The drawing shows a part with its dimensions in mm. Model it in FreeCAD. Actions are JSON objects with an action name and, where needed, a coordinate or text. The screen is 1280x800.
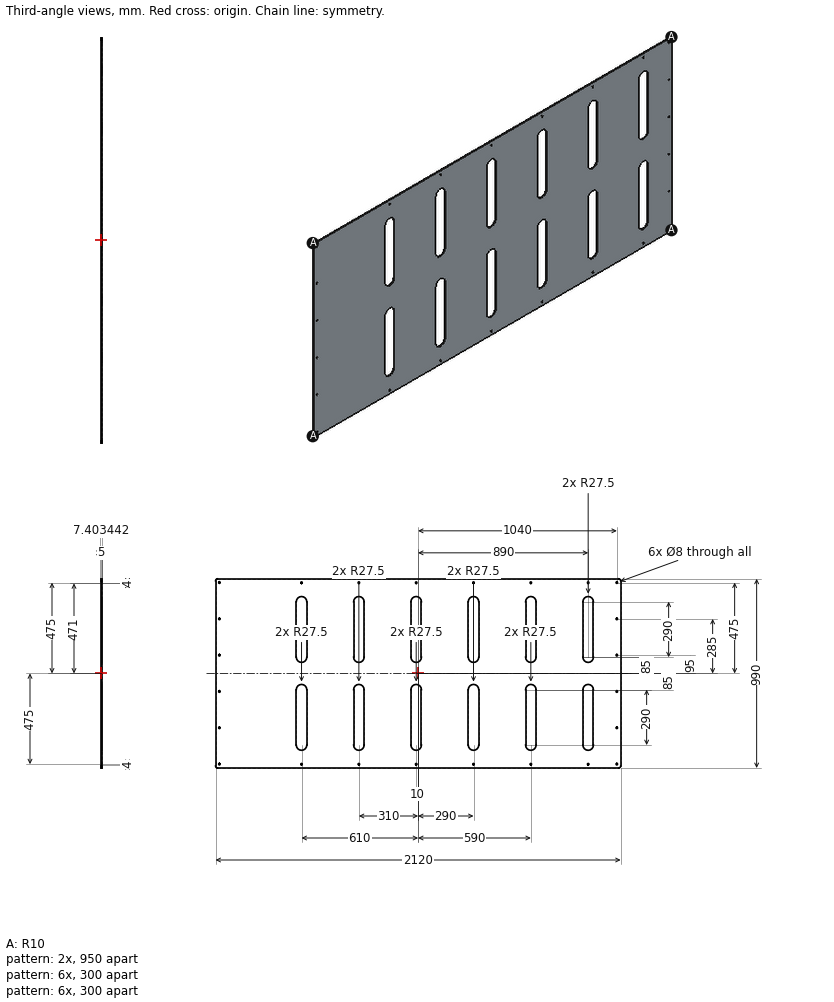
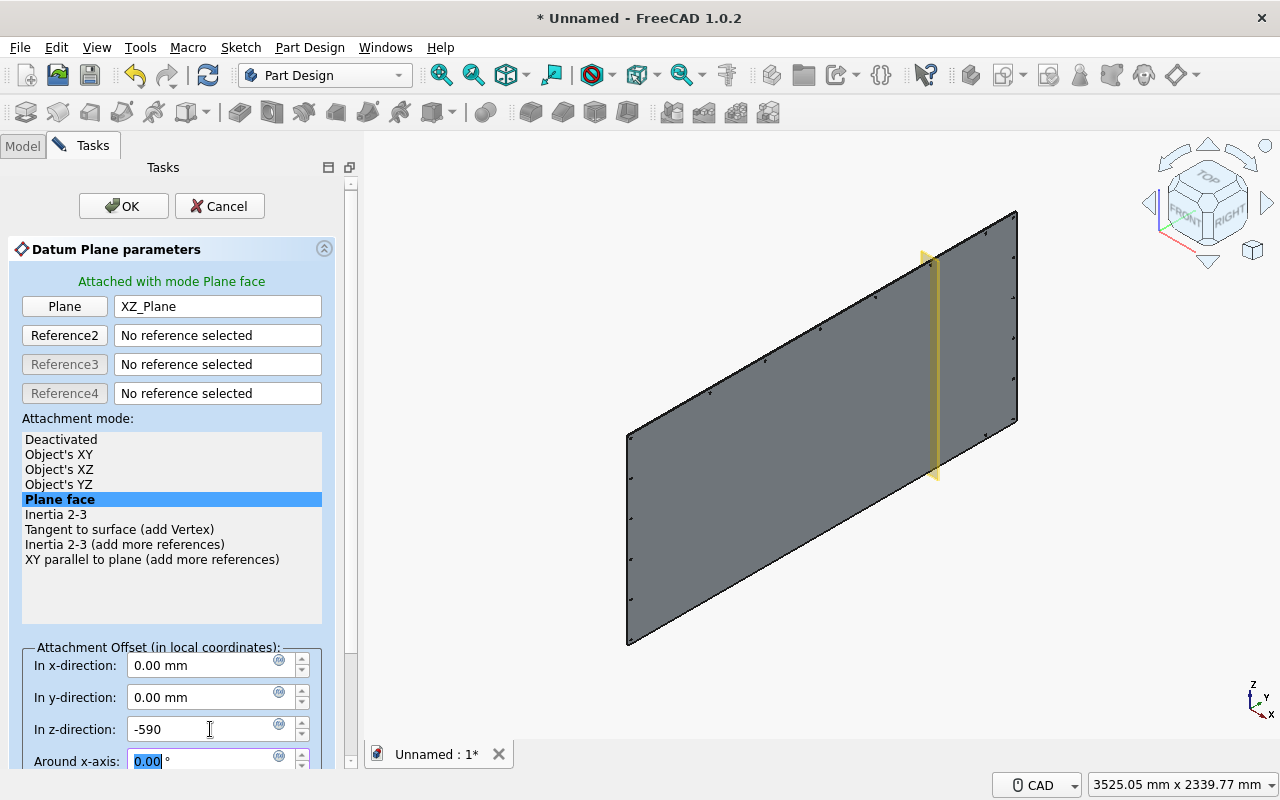
{"action": "left_click", "coordinate": [124, 206]}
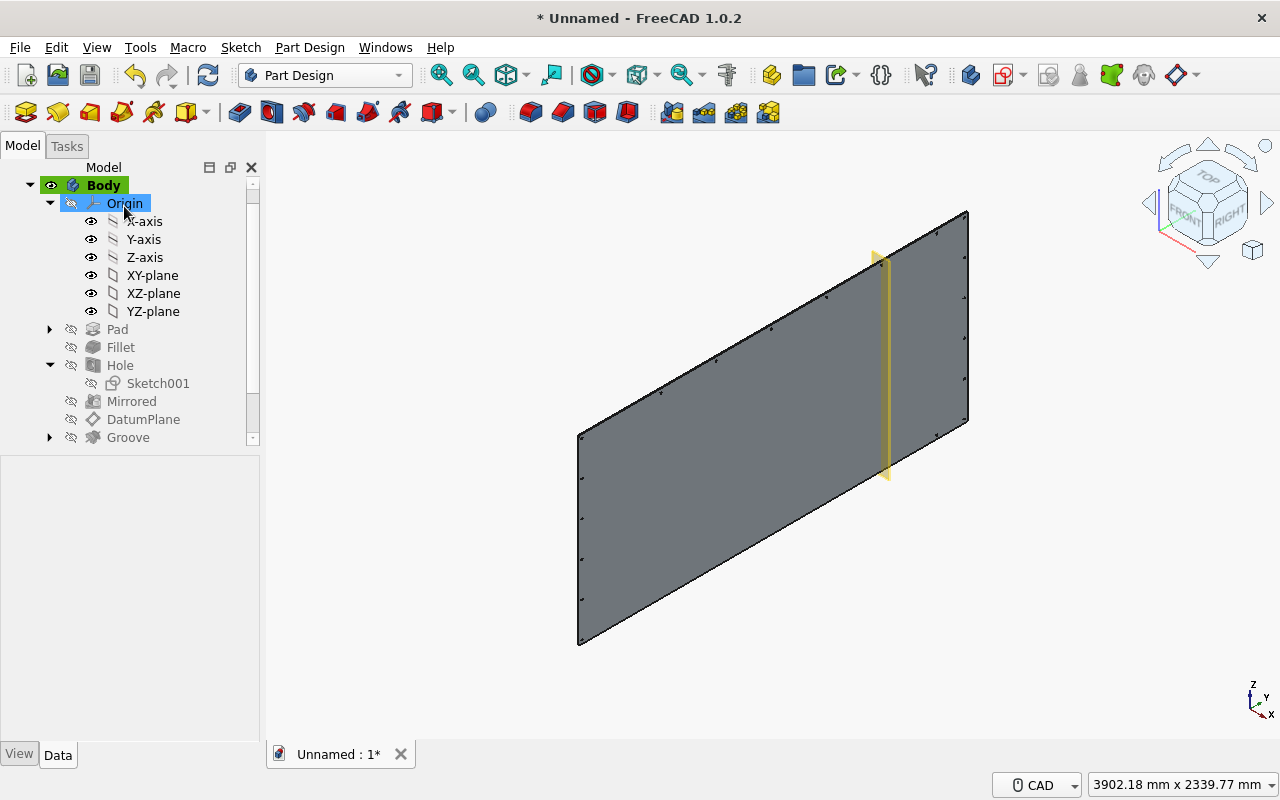
{"action": "scroll", "coordinate": [120, 307], "scroll_direction": "down", "scroll_amount": 3}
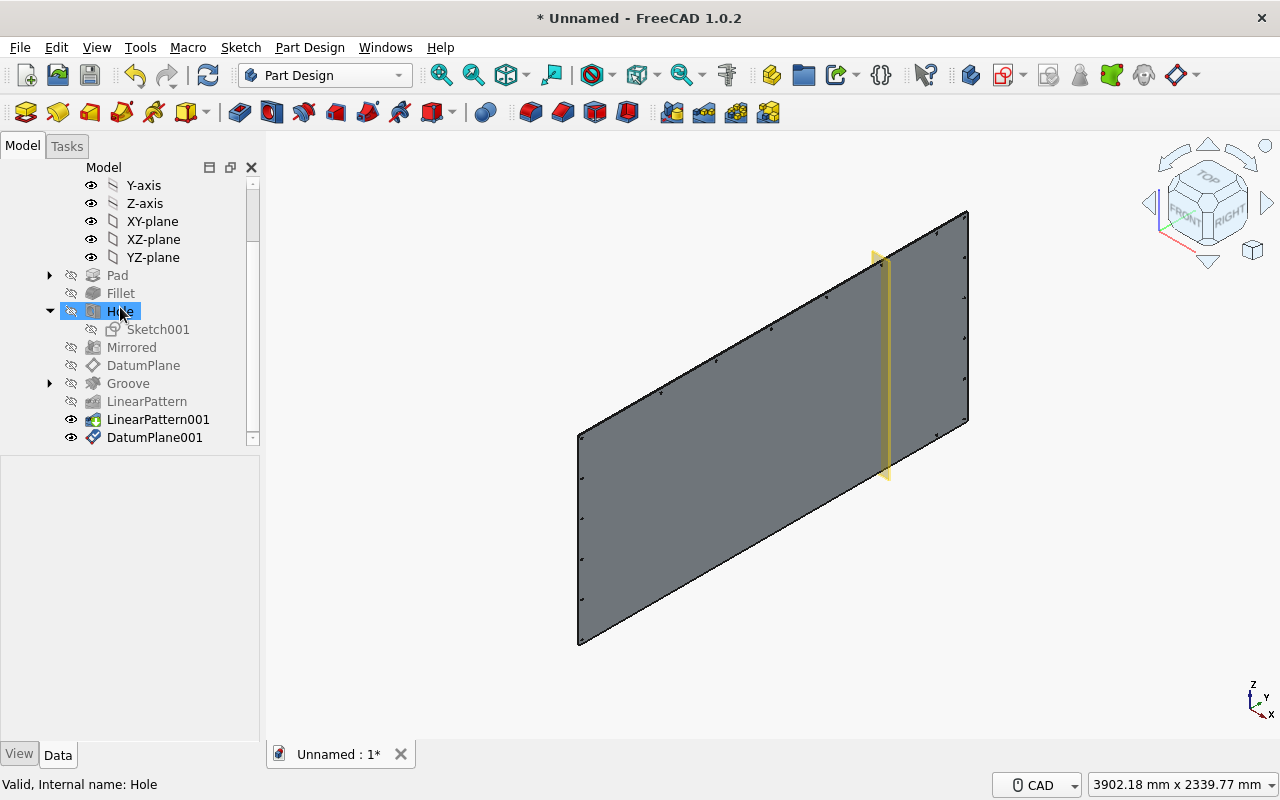
{"action": "left_click", "coordinate": [116, 437]}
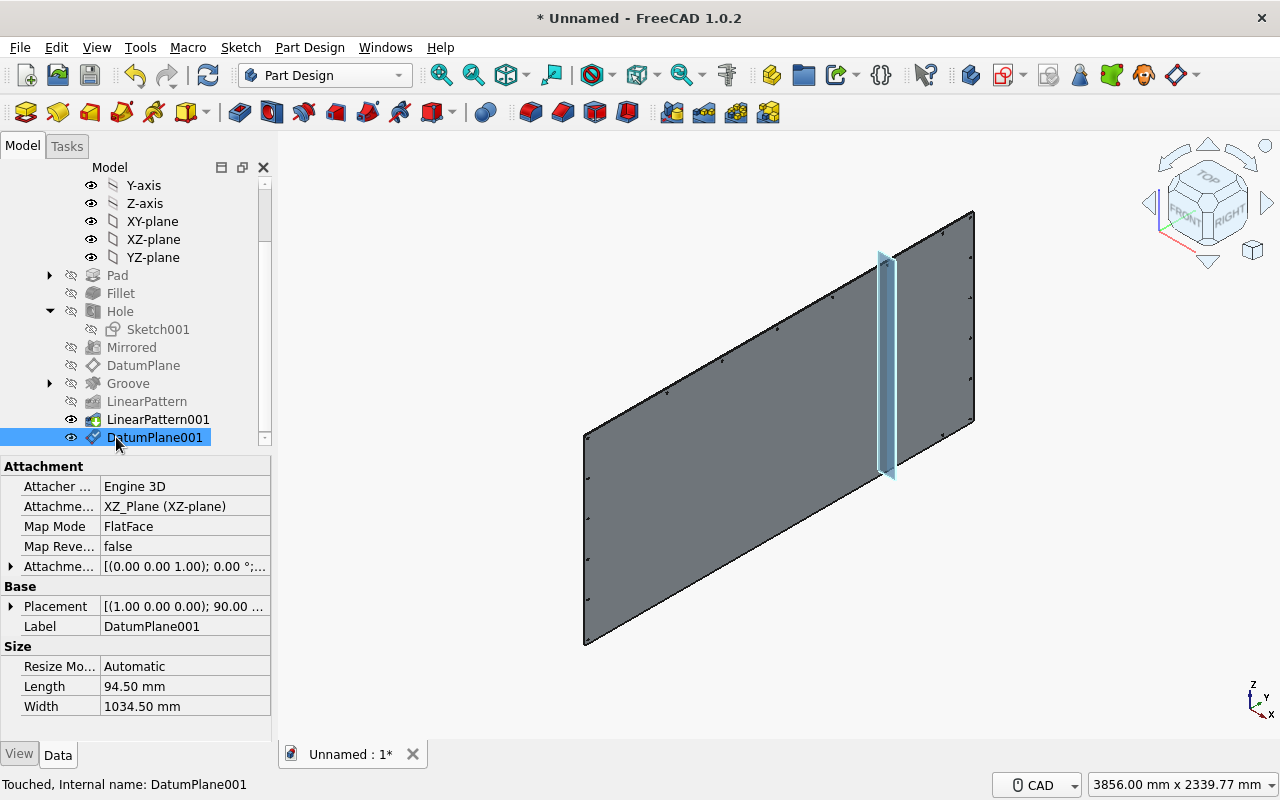
{"action": "left_click", "coordinate": [1004, 76]}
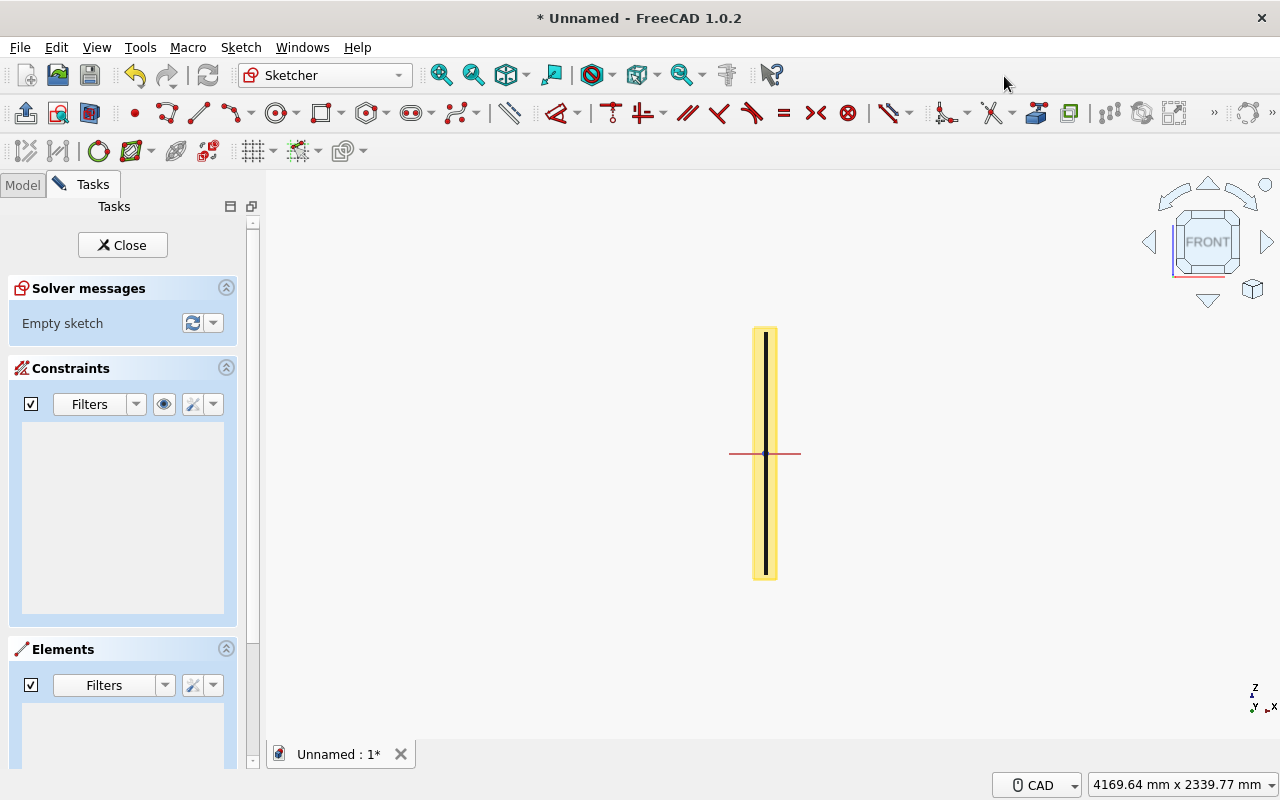
{"action": "left_click", "coordinate": [90, 114]}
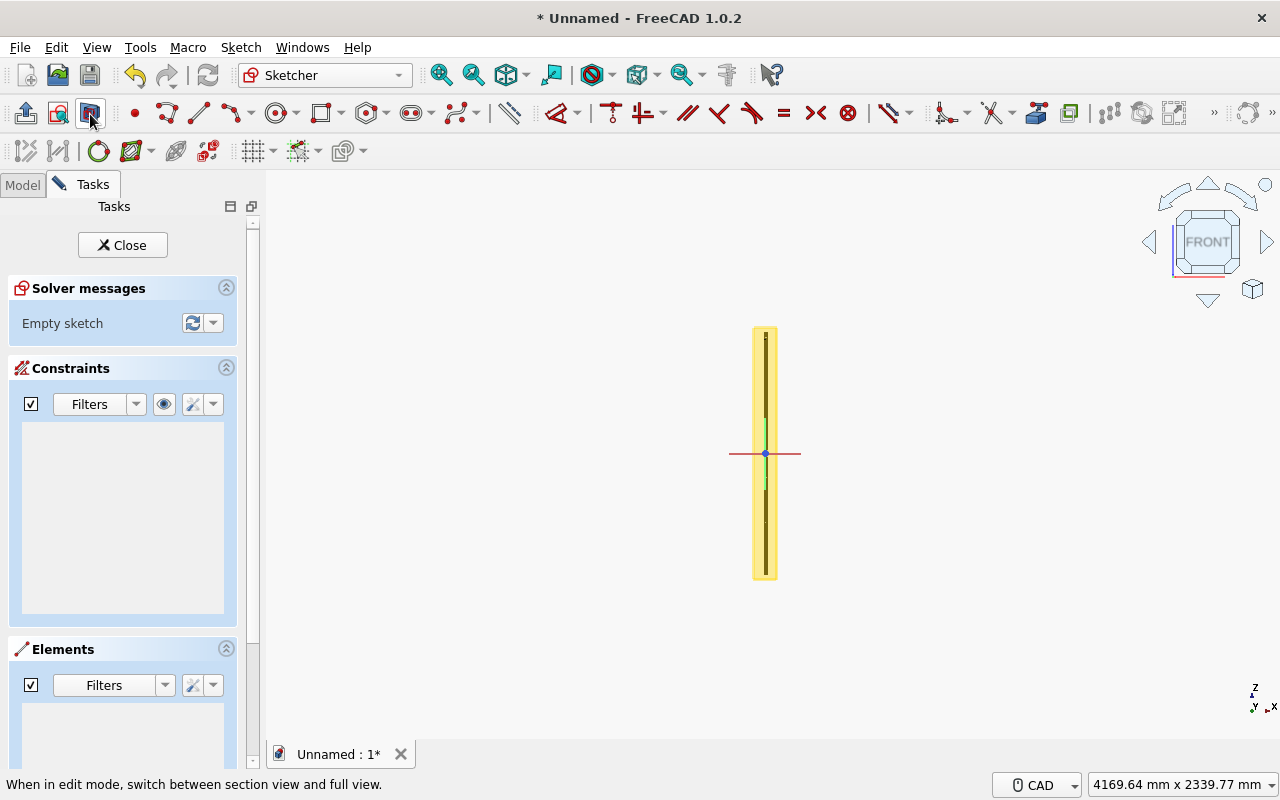
{"action": "scroll", "coordinate": [769, 576], "scroll_direction": "up", "scroll_amount": 15}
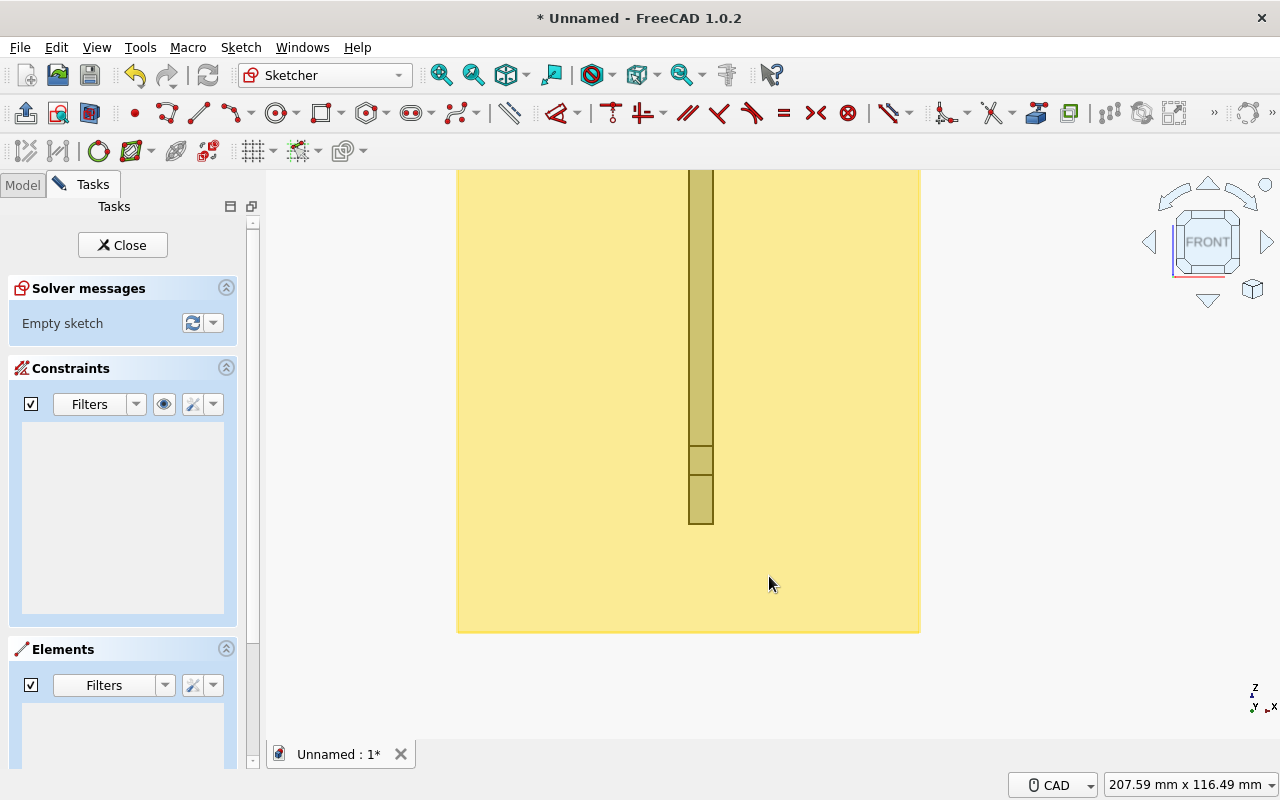
{"action": "scroll", "coordinate": [686, 434], "scroll_direction": "up", "scroll_amount": 12}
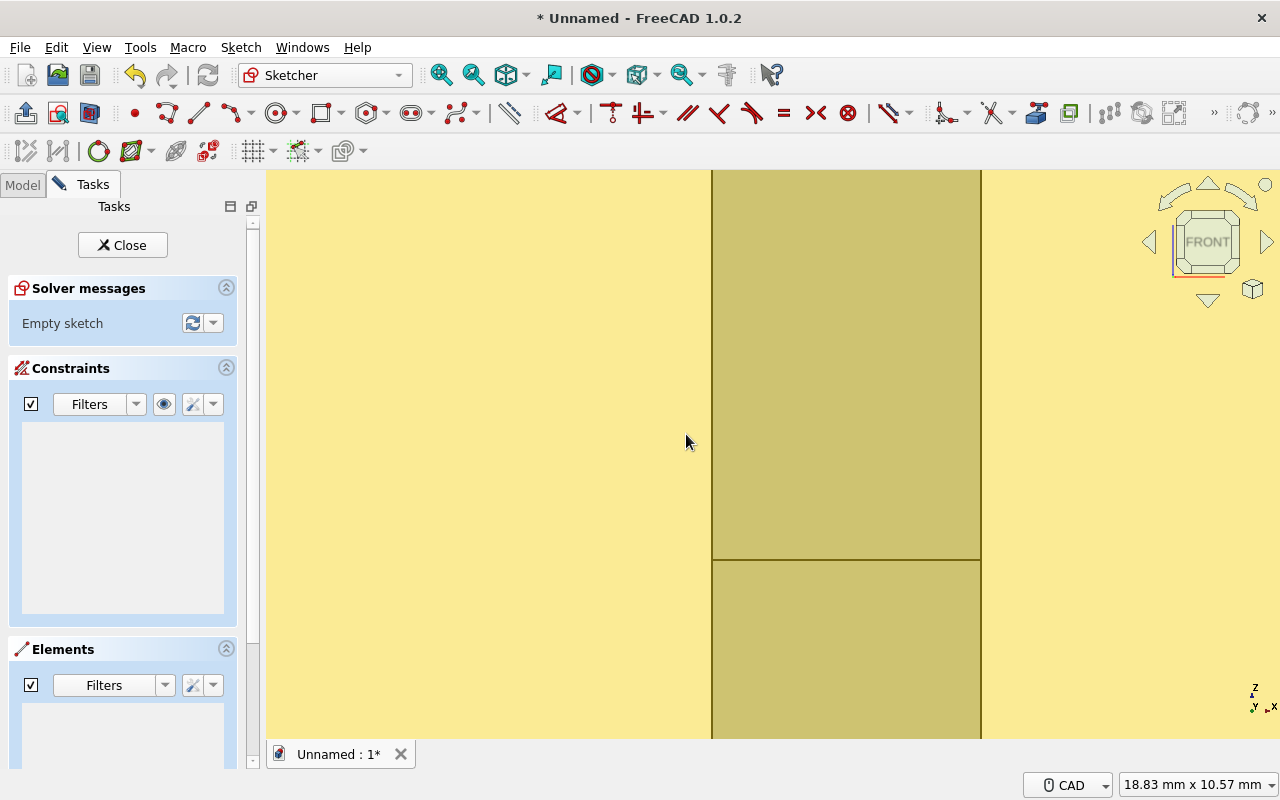
{"action": "left_click", "coordinate": [168, 114]}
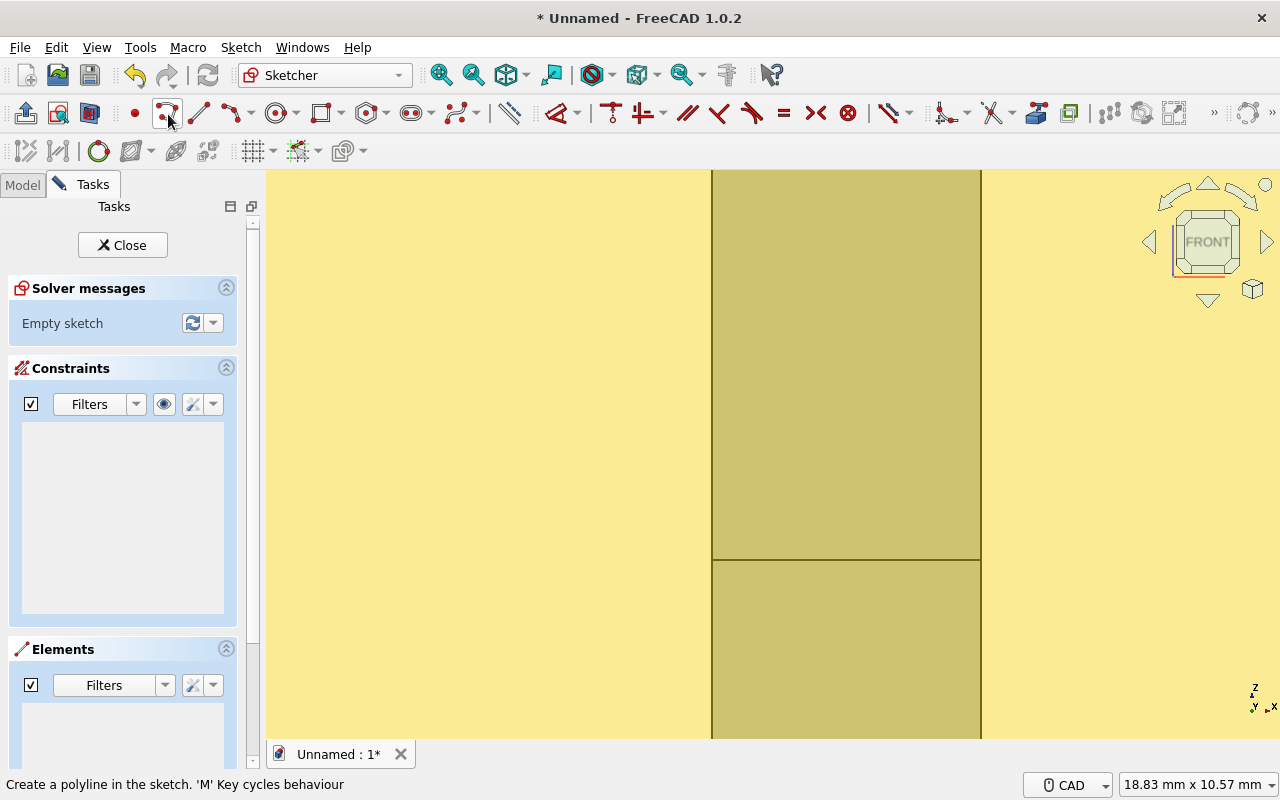
{"action": "left_click", "coordinate": [582, 345]}
{"action": "left_click", "coordinate": [981, 345]}
{"action": "left_click", "coordinate": [981, 560]}
{"action": "left_click", "coordinate": [712, 560]}
{"action": "left_click", "coordinate": [582, 346]}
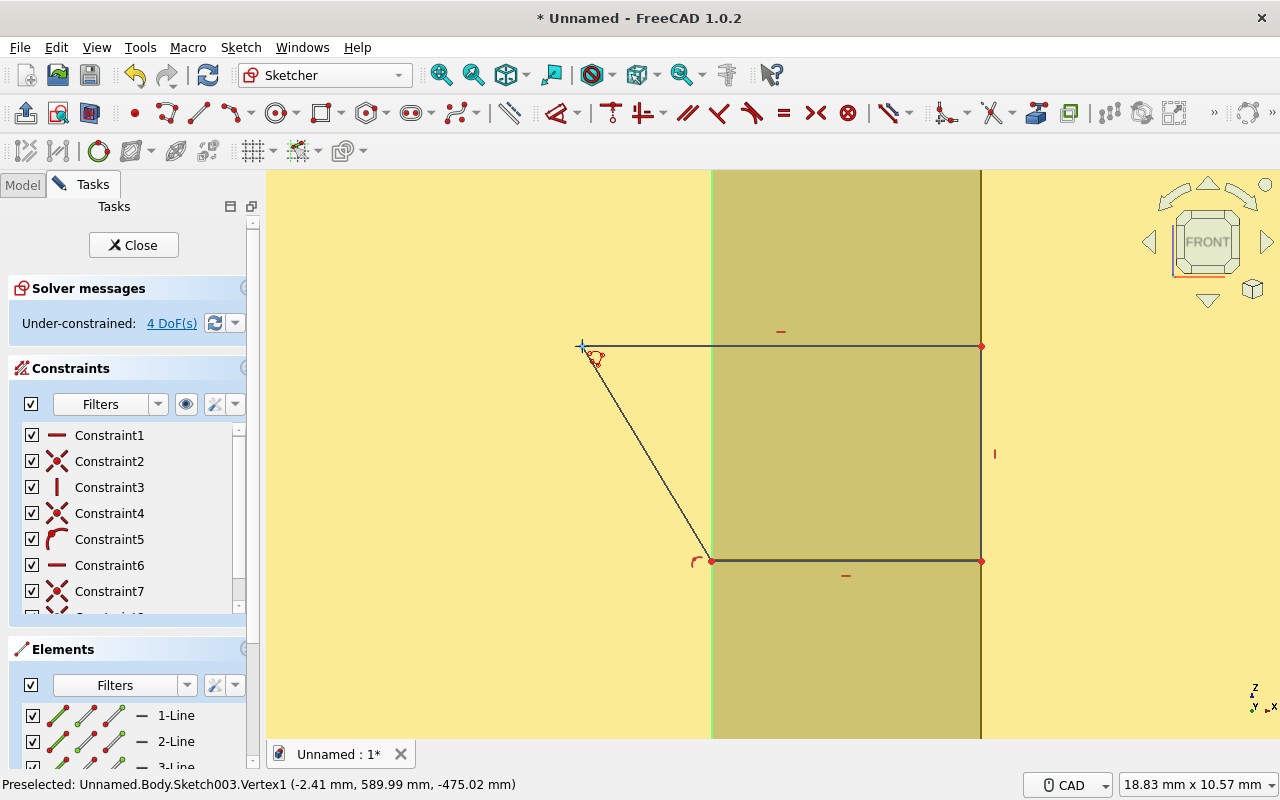
{"action": "left_click", "coordinate": [200, 114]}